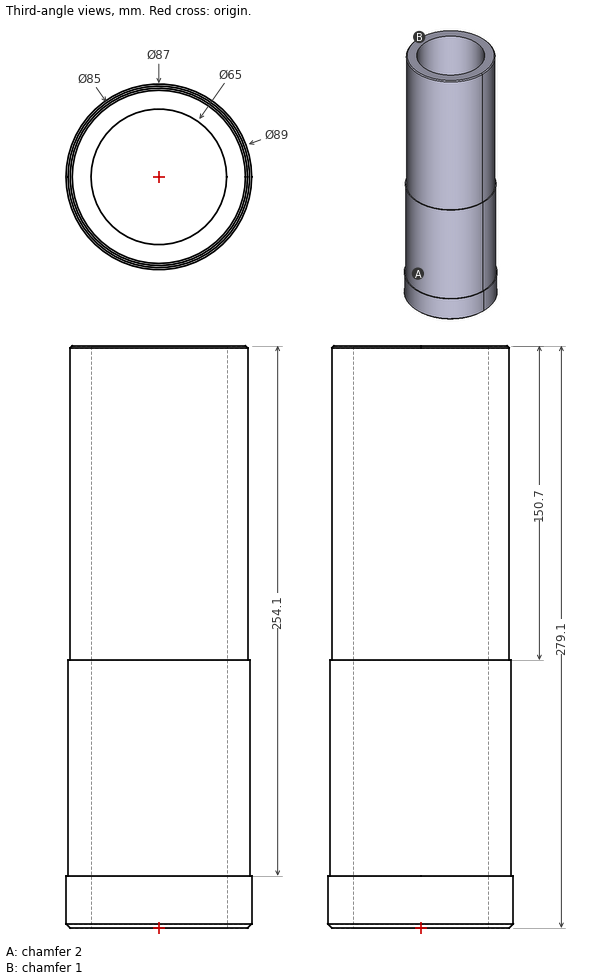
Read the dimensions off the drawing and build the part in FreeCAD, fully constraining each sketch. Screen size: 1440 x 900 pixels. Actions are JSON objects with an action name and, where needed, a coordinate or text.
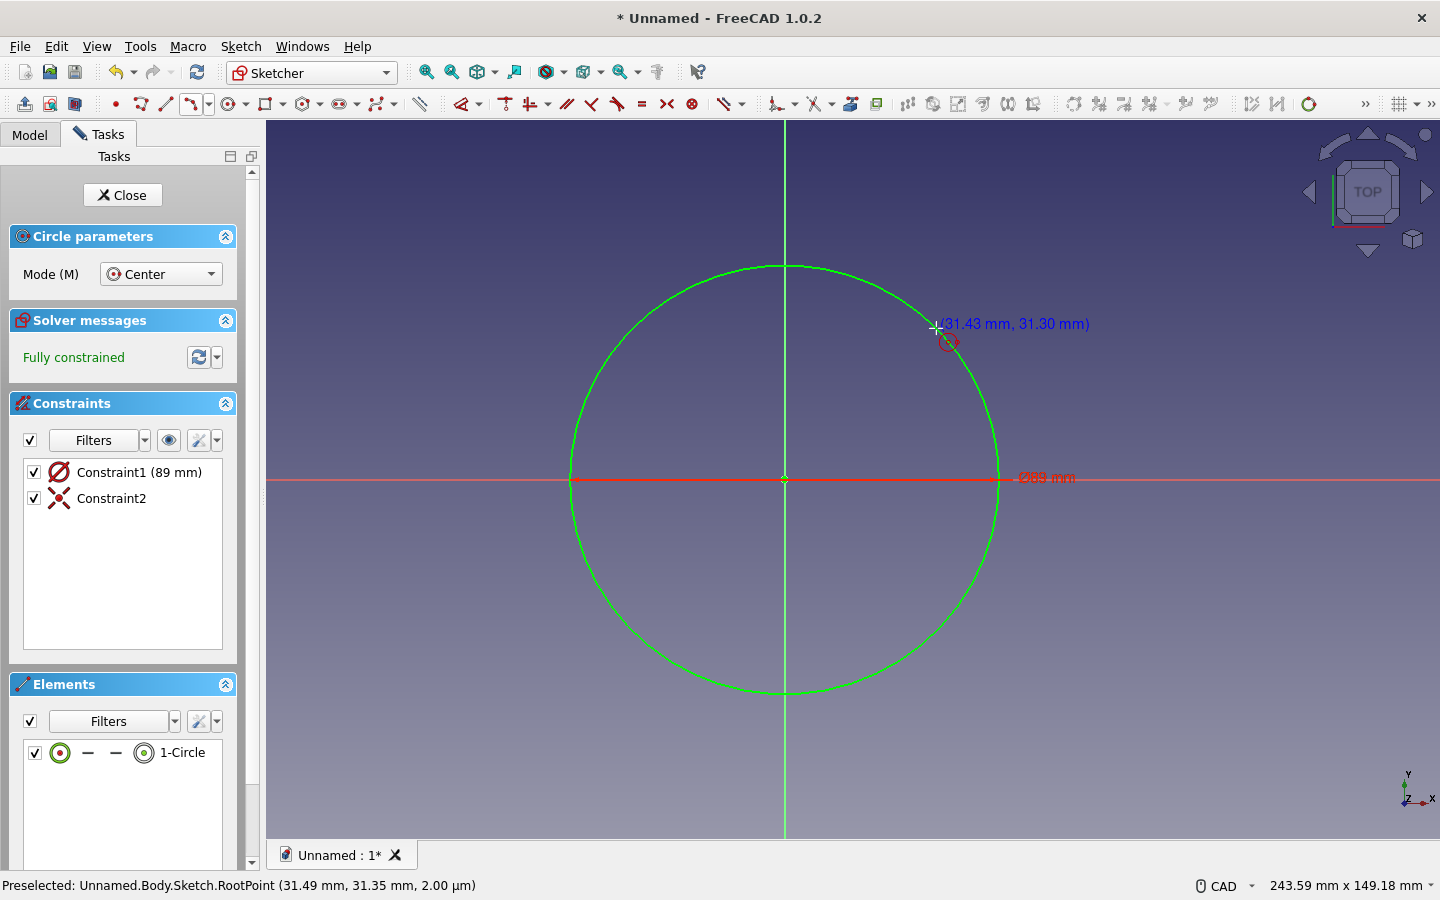
{"action": "left_click", "coordinate": [785, 480]}
{"action": "mouse_move", "coordinate": [895, 369]}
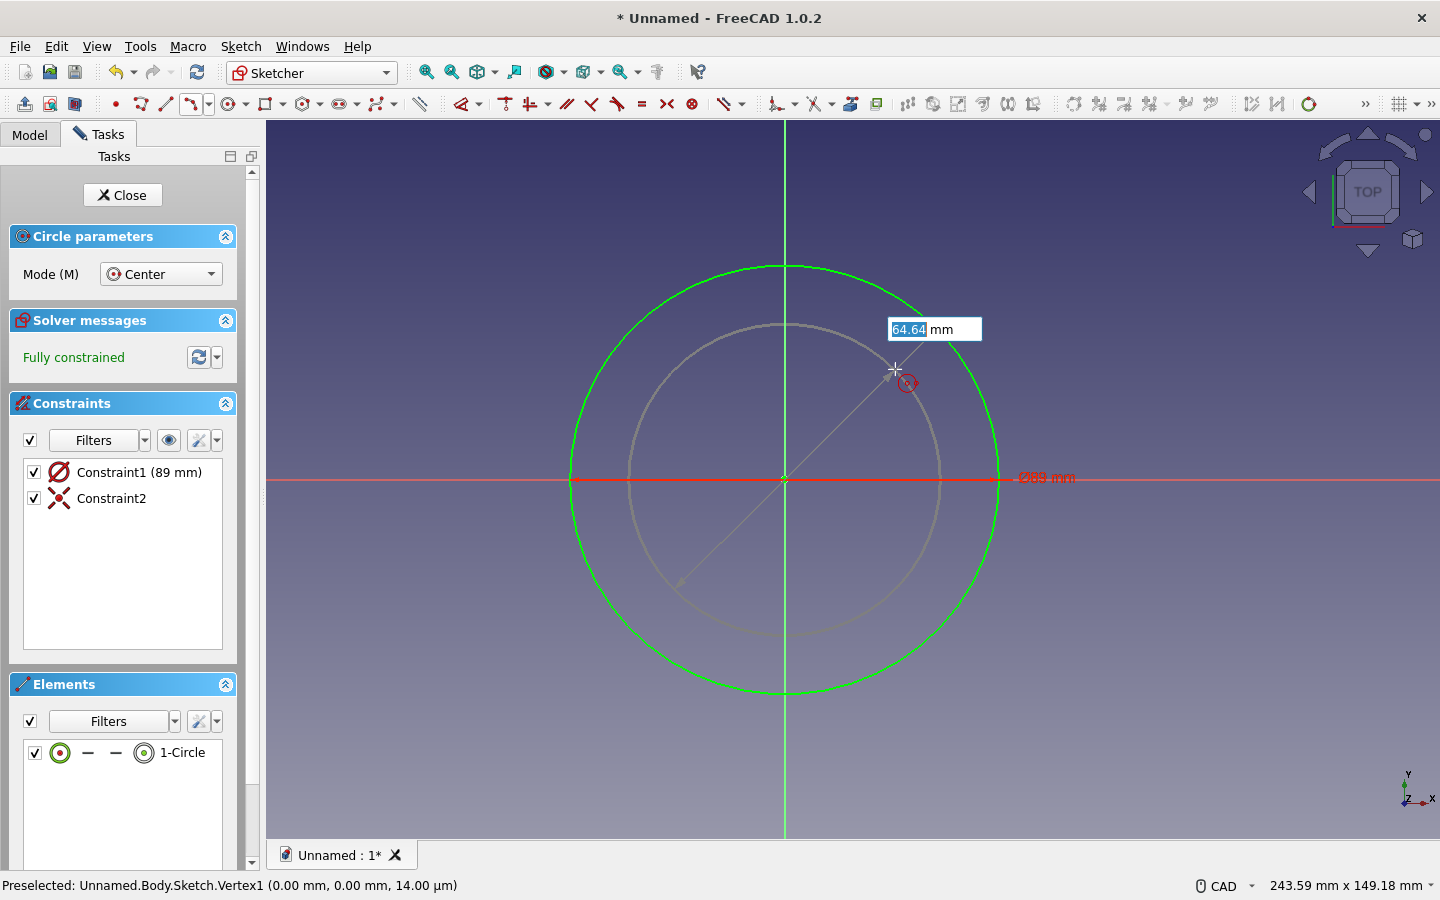
{"action": "type", "text": "65"}
{"action": "key", "text": "Return"}
{"action": "key", "text": "Escape"}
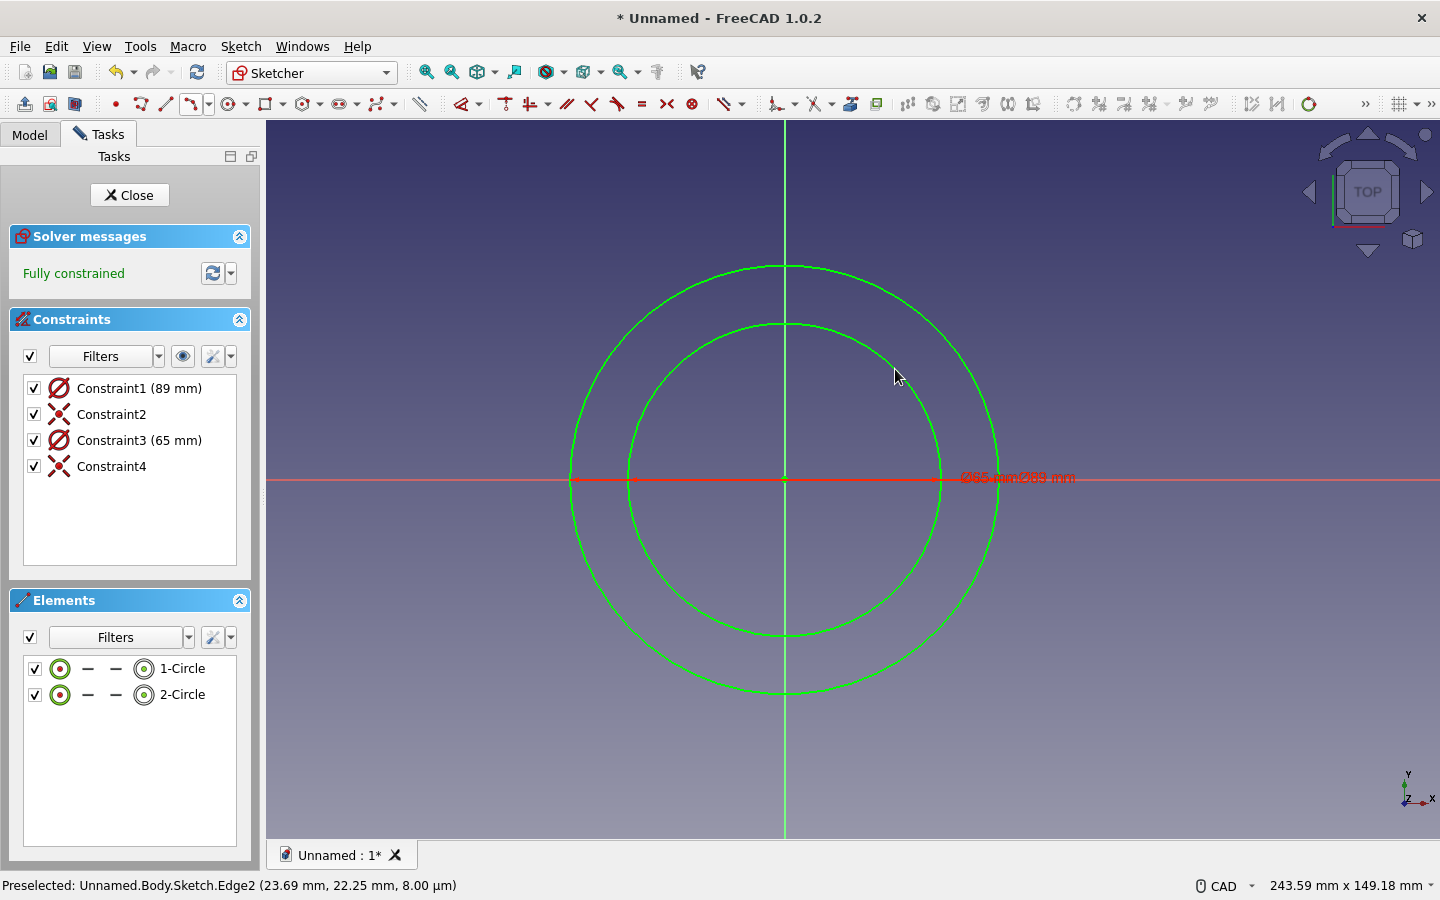
{"action": "left_click", "coordinate": [130, 195]}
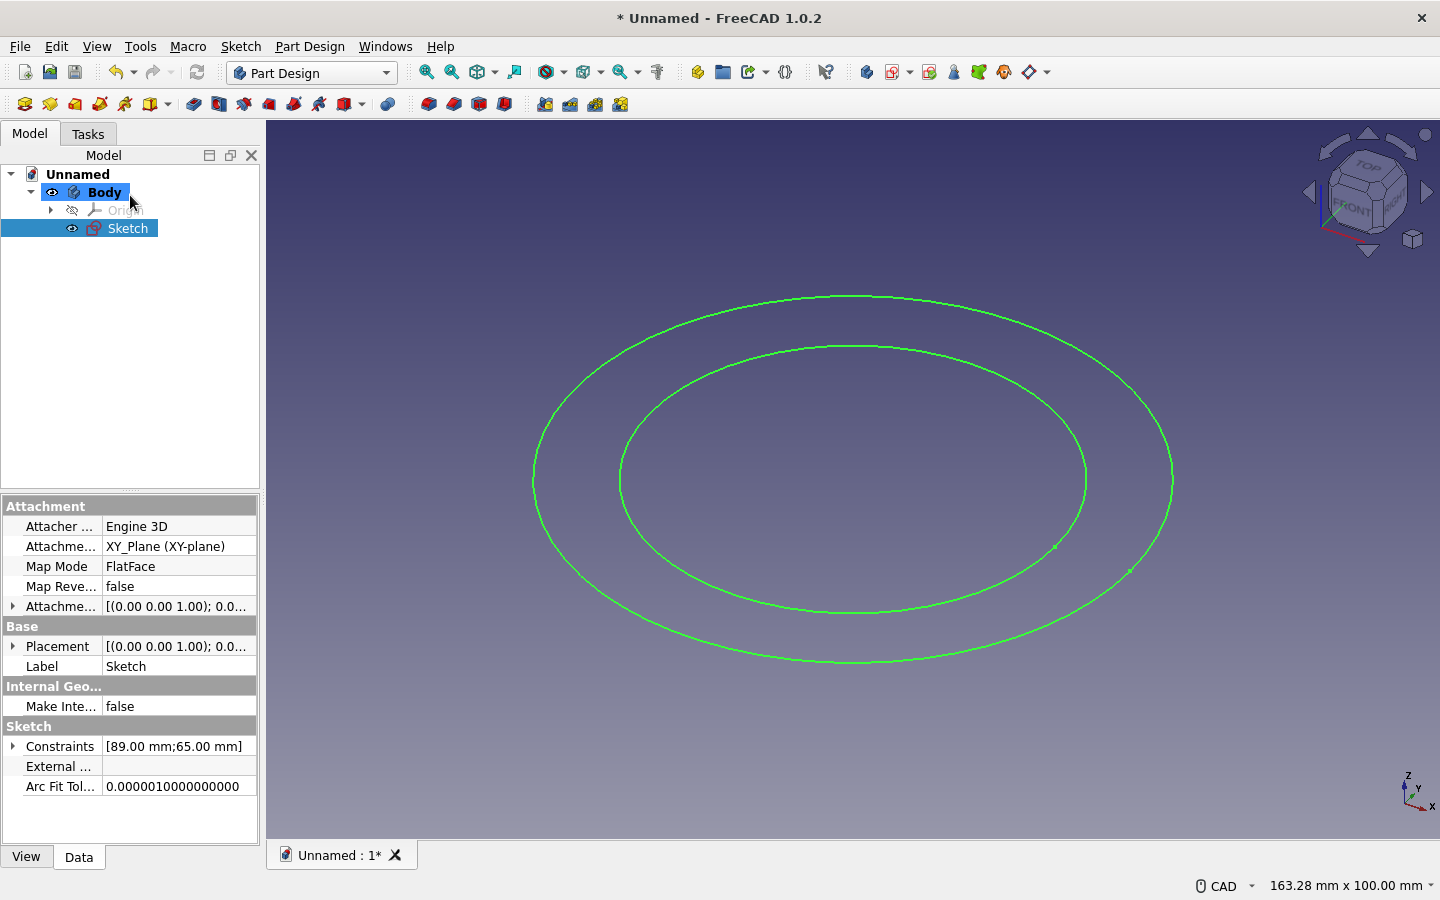
{"action": "left_click", "coordinate": [25, 104]}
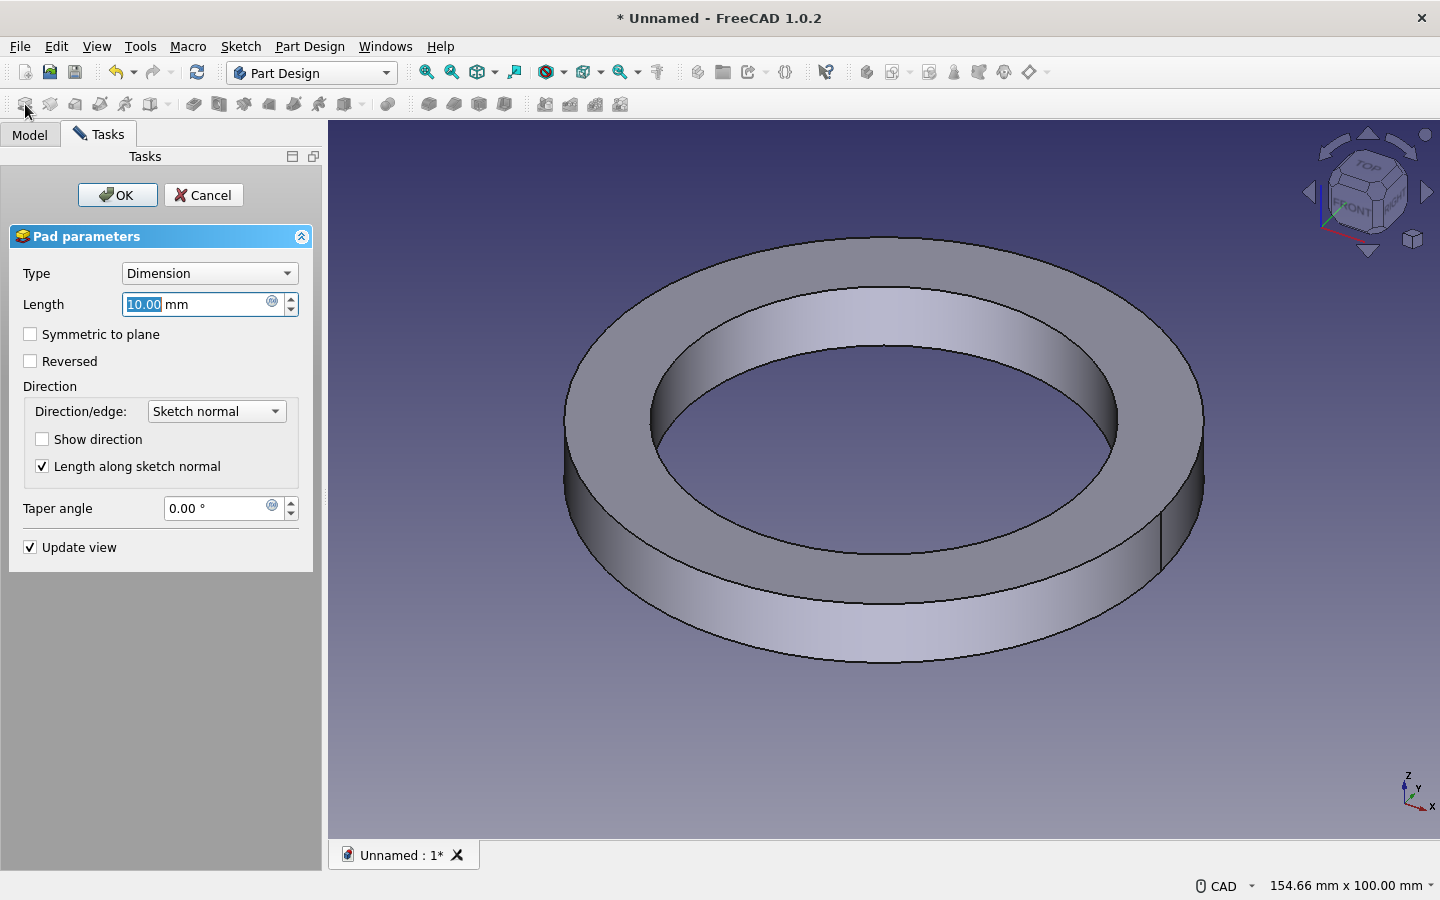
{"action": "type", "text": "279.1"}
{"action": "key", "text": "Tab"}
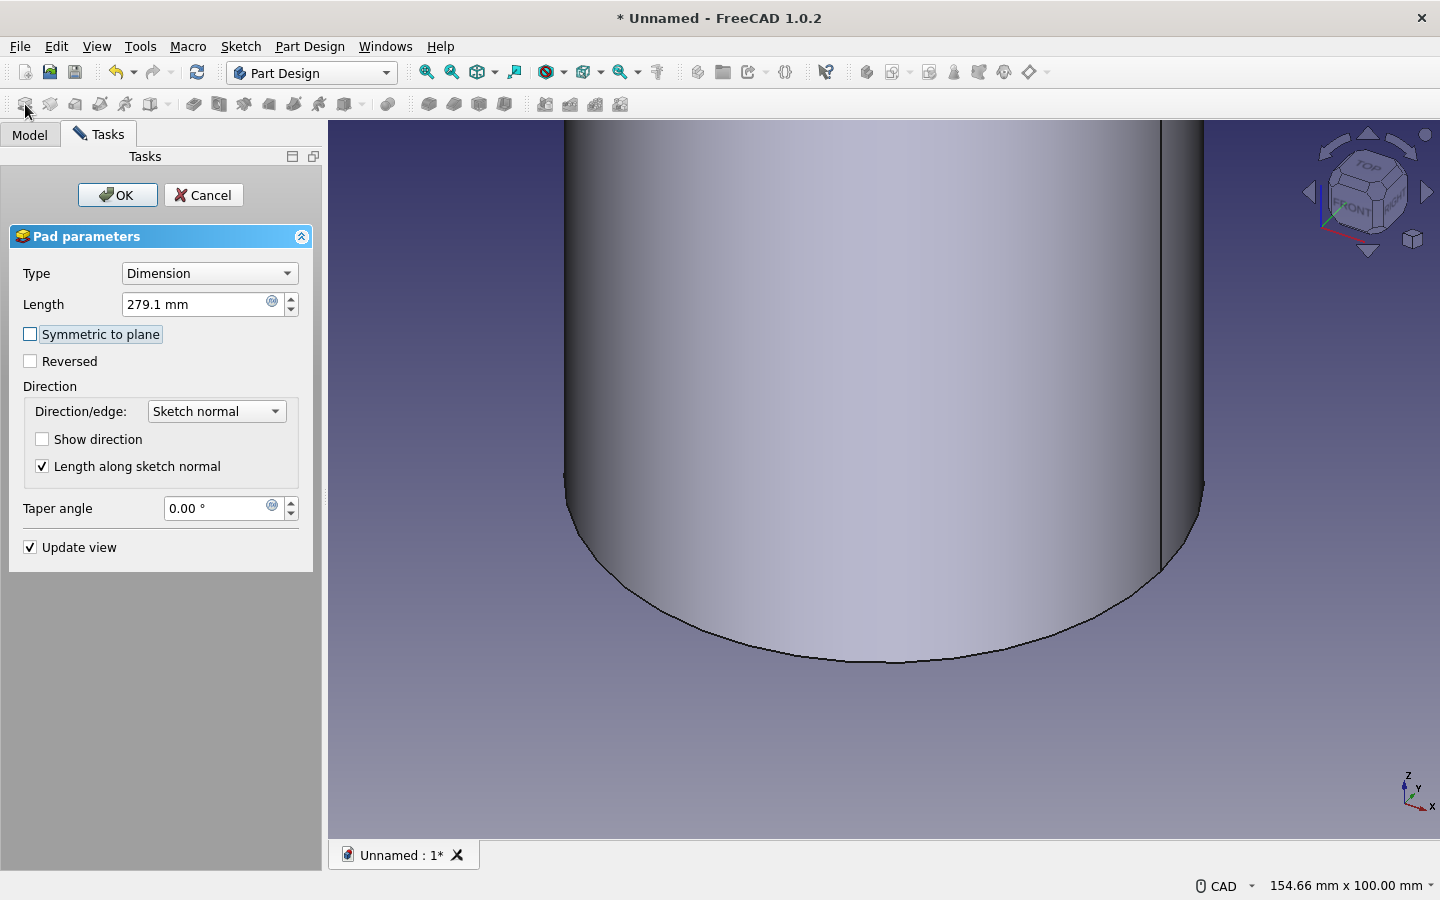
{"action": "left_click", "coordinate": [118, 195]}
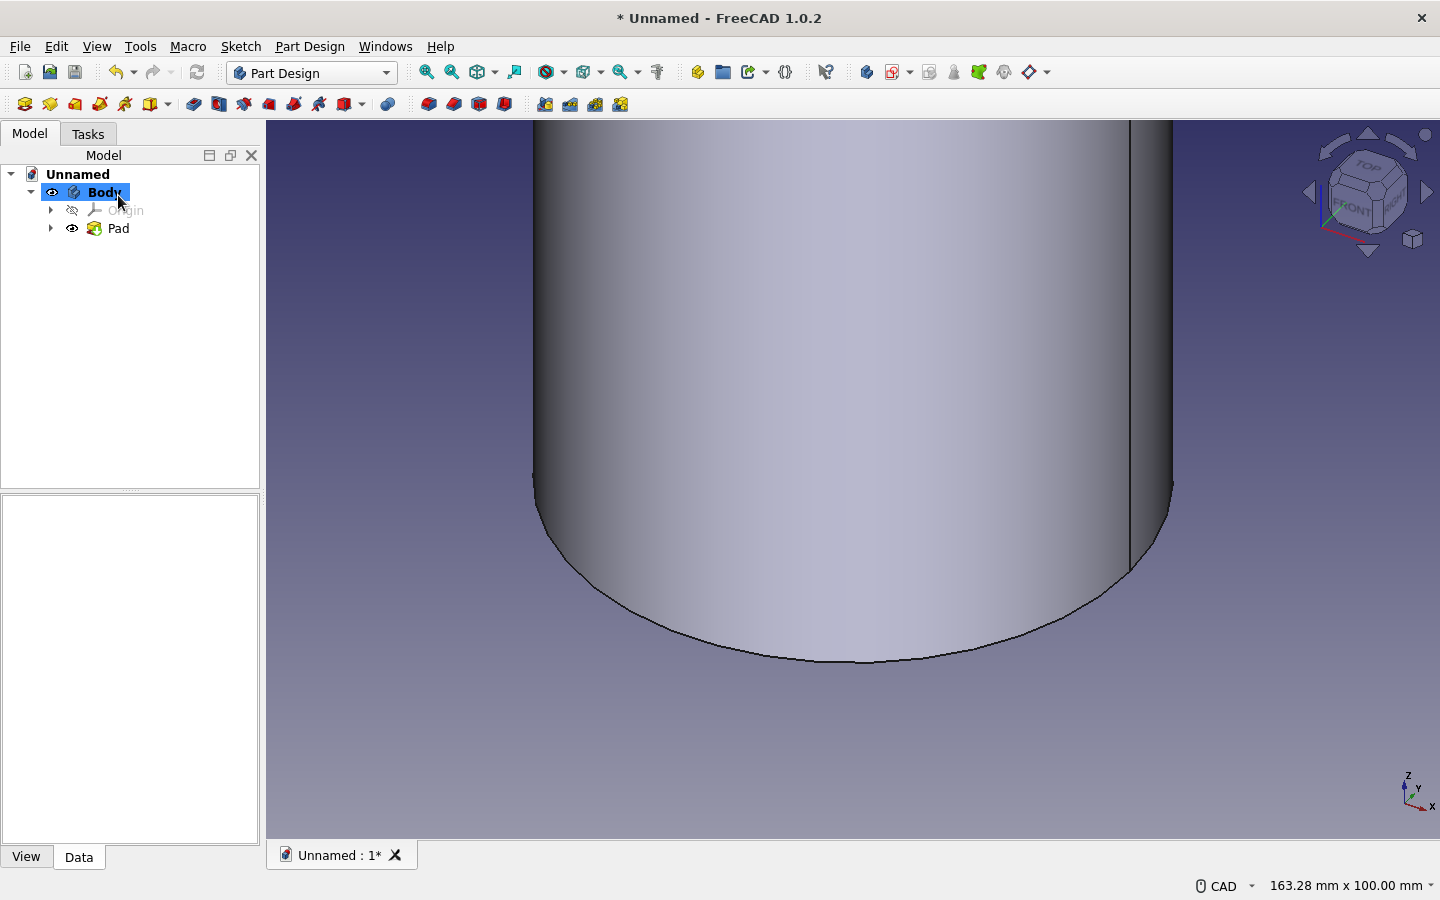
{"action": "left_click", "coordinate": [427, 72]}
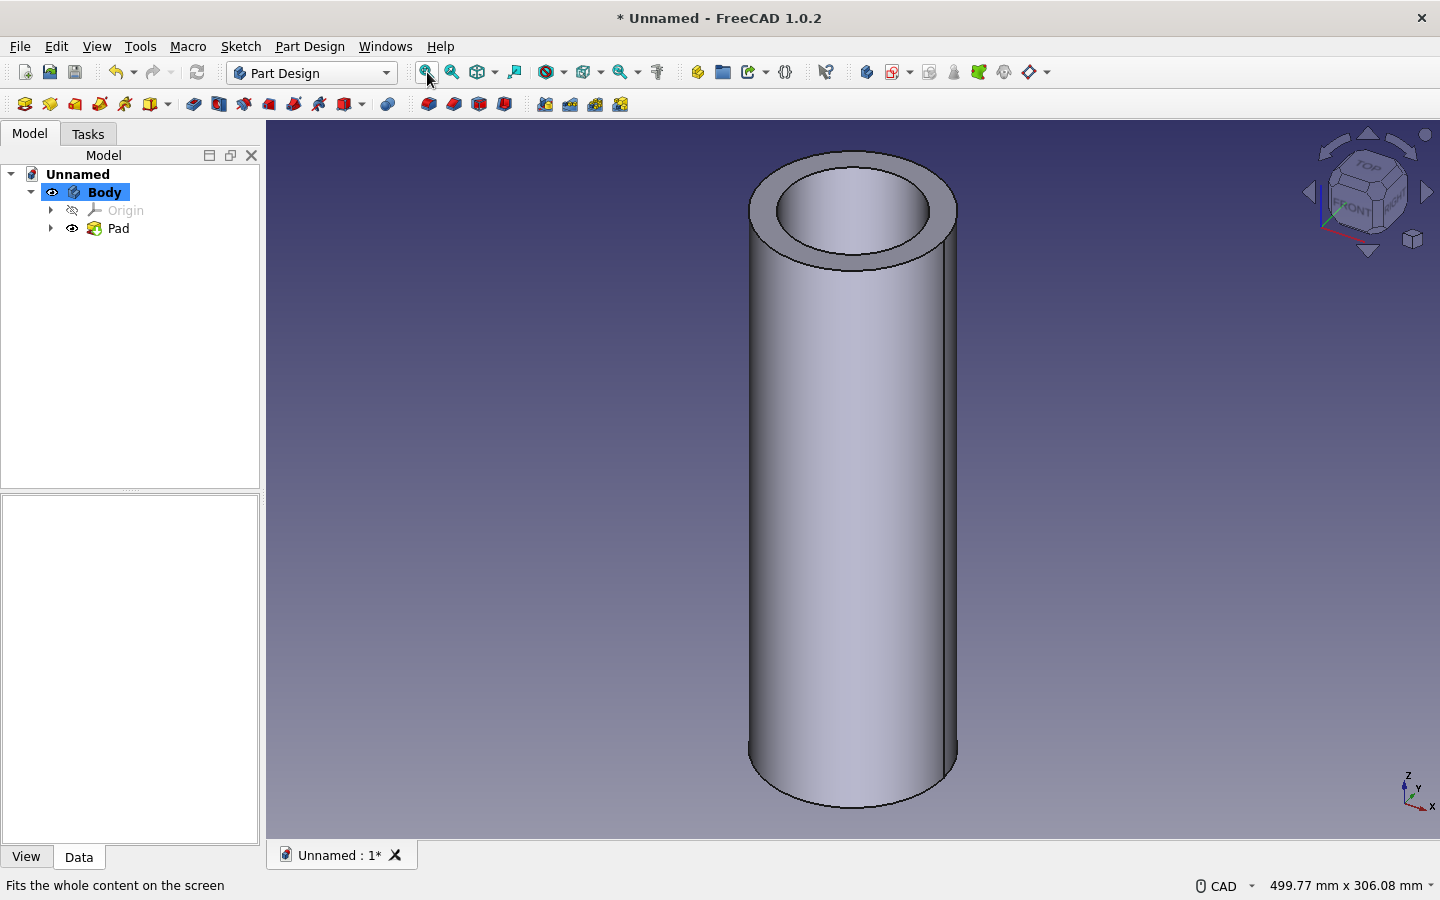
{"action": "left_click", "coordinate": [51, 210]}